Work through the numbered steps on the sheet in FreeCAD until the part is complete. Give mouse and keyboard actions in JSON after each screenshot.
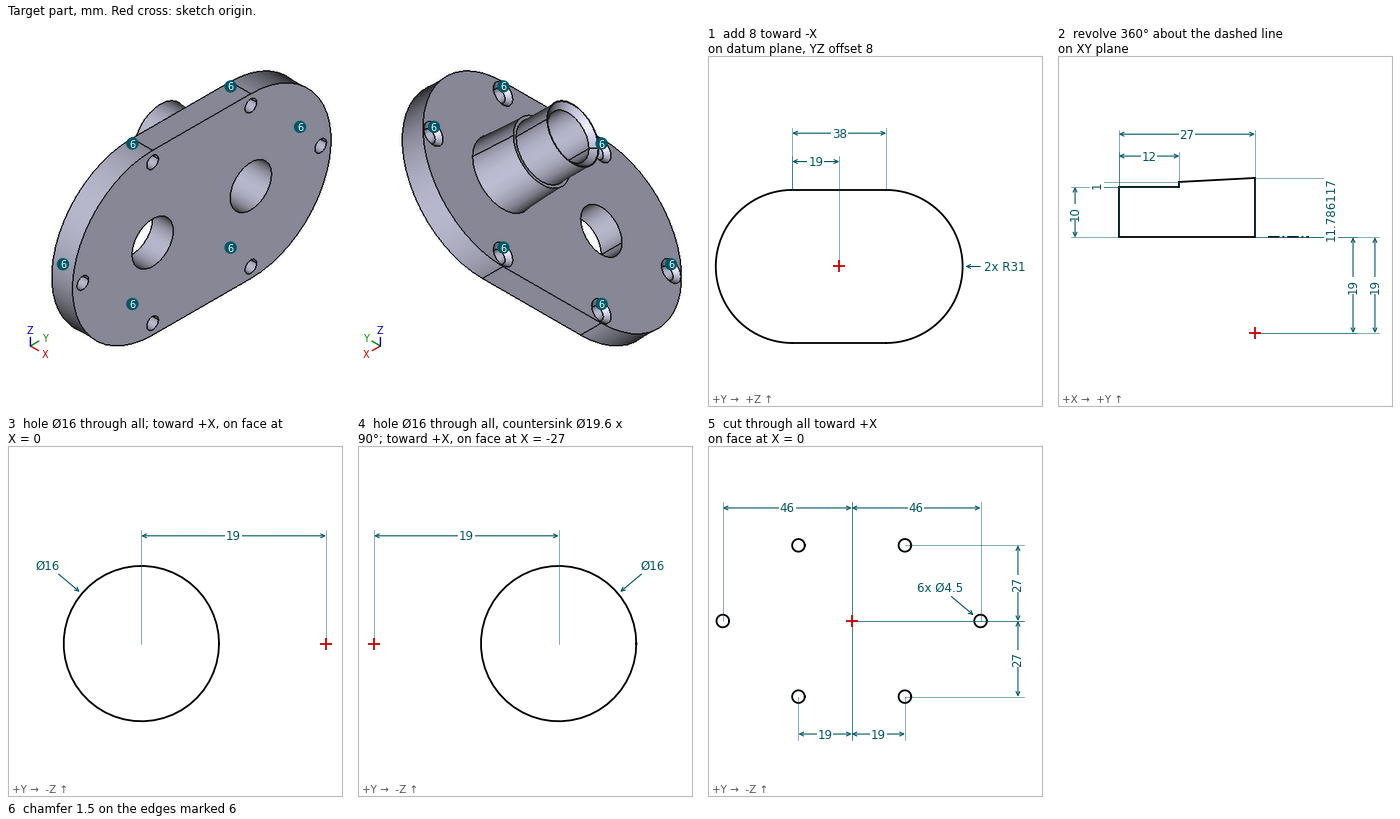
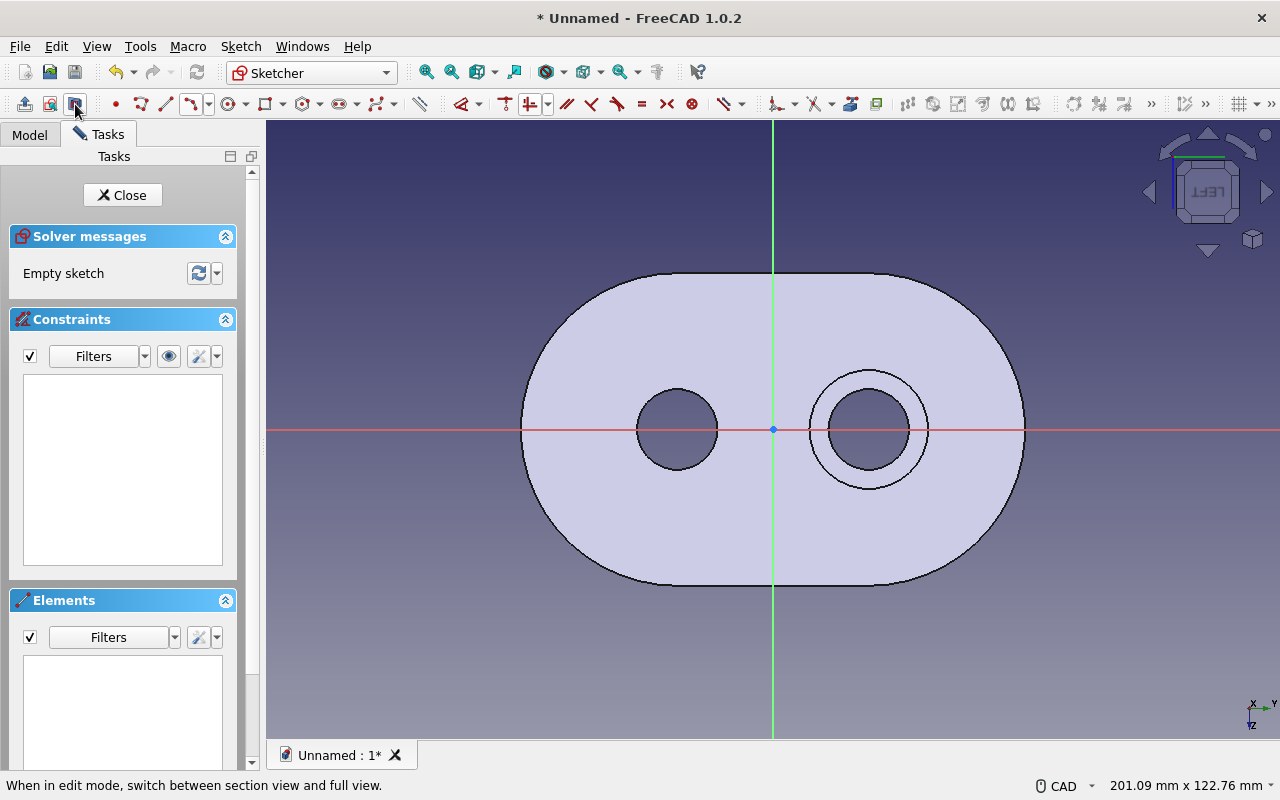
{"action": "left_click", "coordinate": [228, 104]}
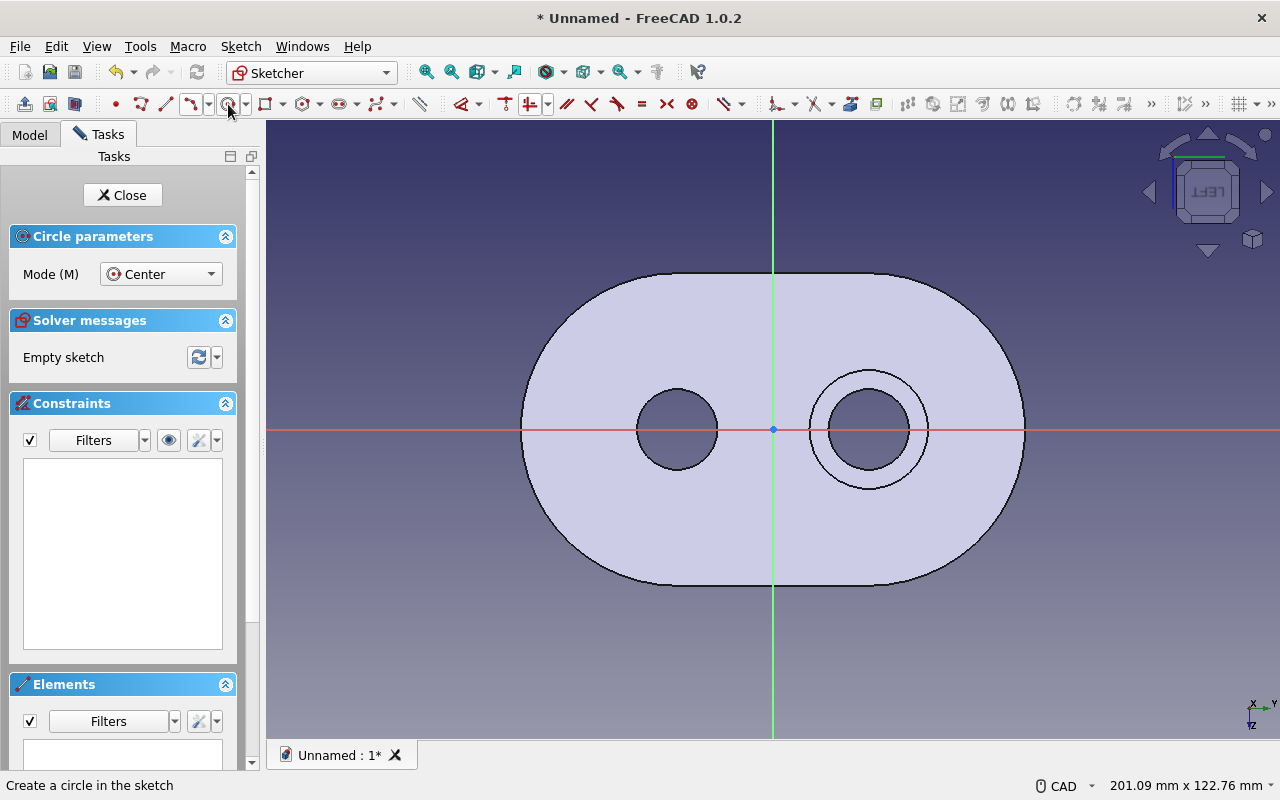
{"action": "scroll", "coordinate": [1005, 429], "scroll_direction": "up", "scroll_amount": 4}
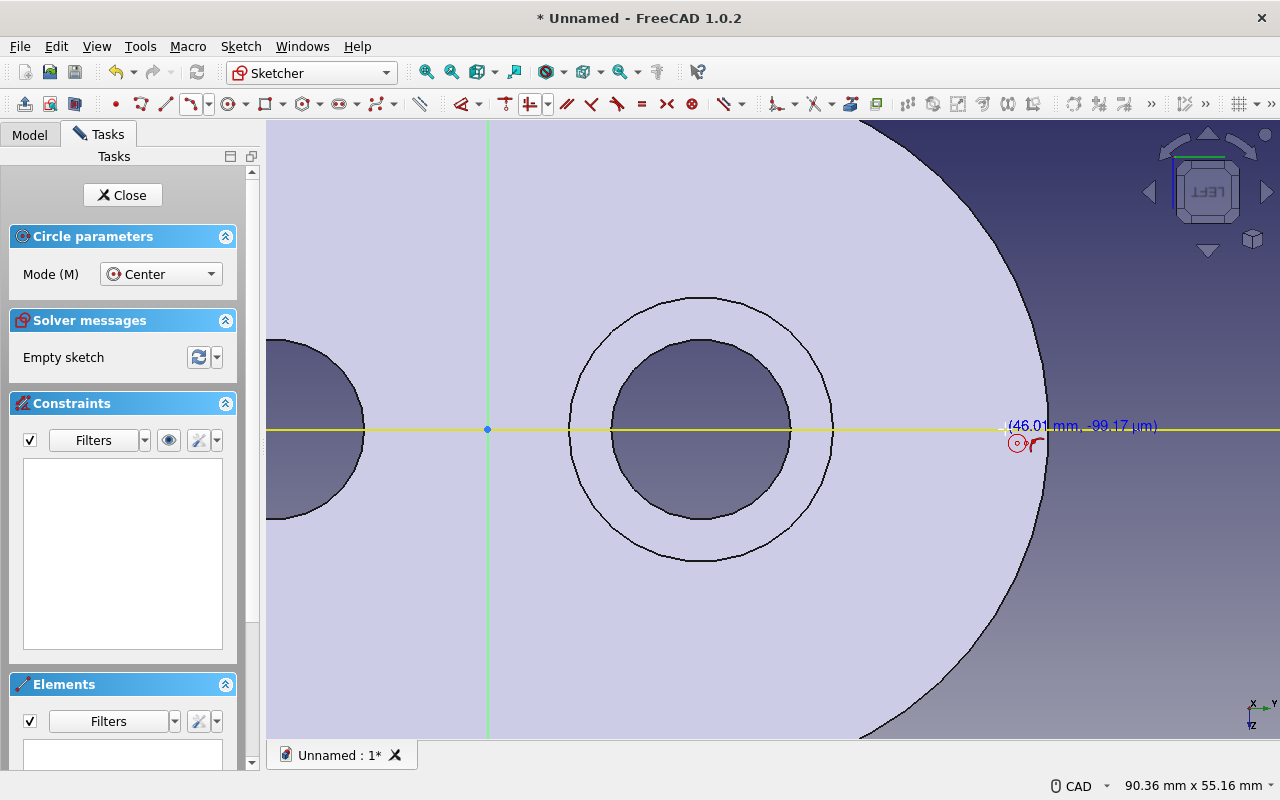
{"action": "left_click", "coordinate": [1004, 429]}
{"action": "left_click", "coordinate": [1022, 412]}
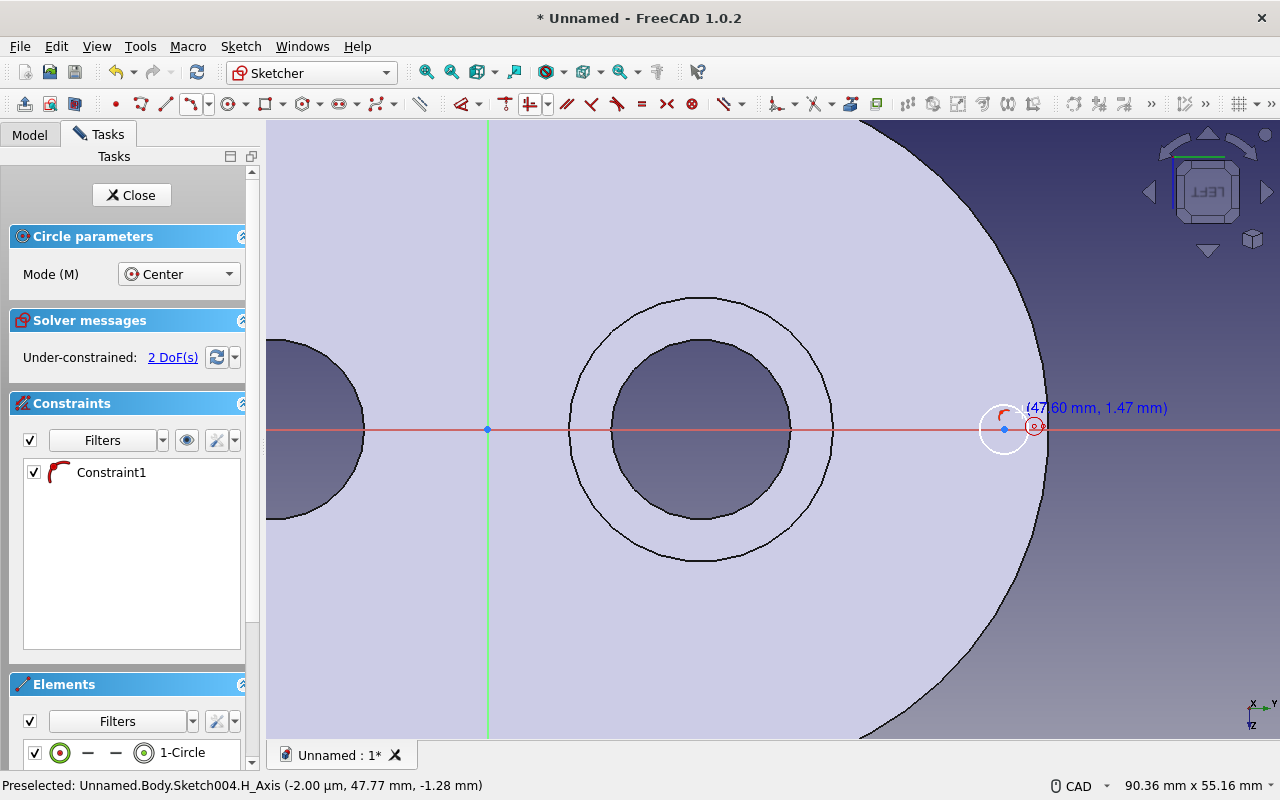
{"action": "scroll", "coordinate": [968, 430], "scroll_direction": "down", "scroll_amount": 3}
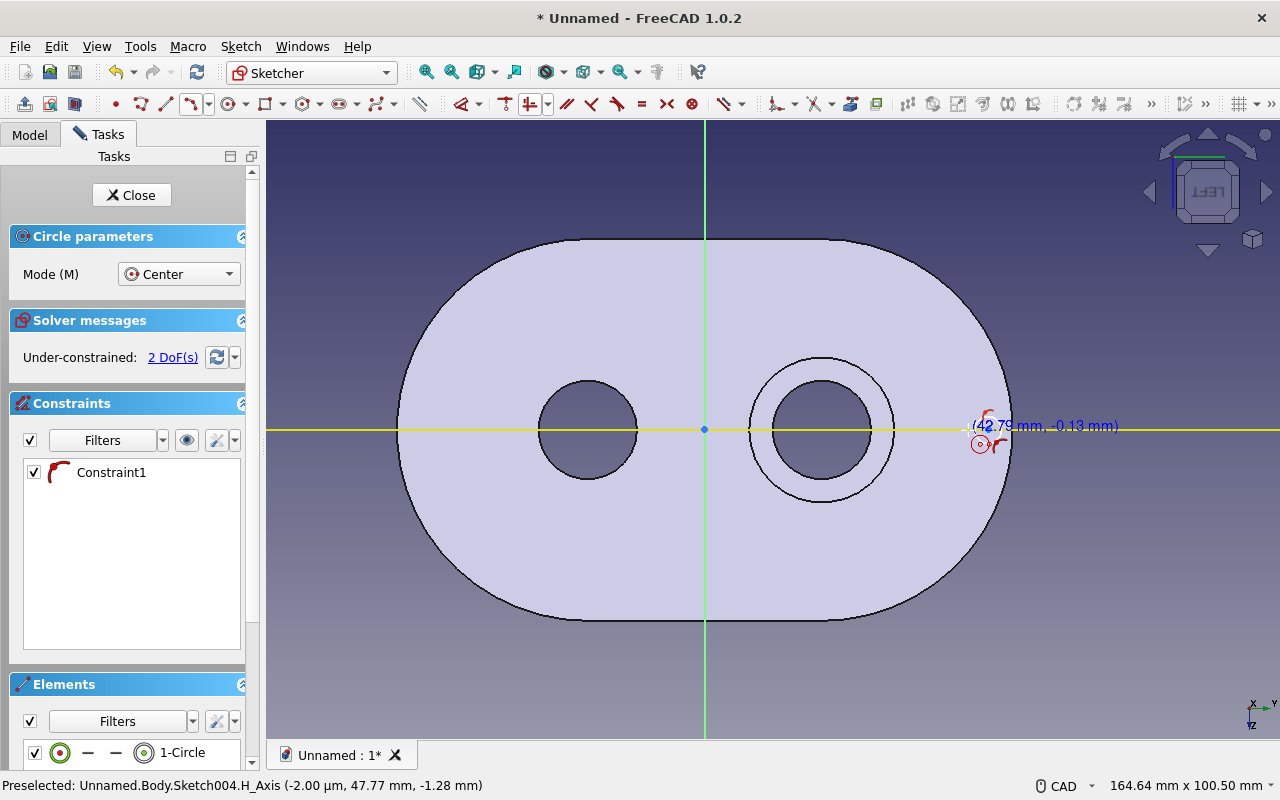
{"action": "scroll", "coordinate": [822, 596], "scroll_direction": "up", "scroll_amount": 3}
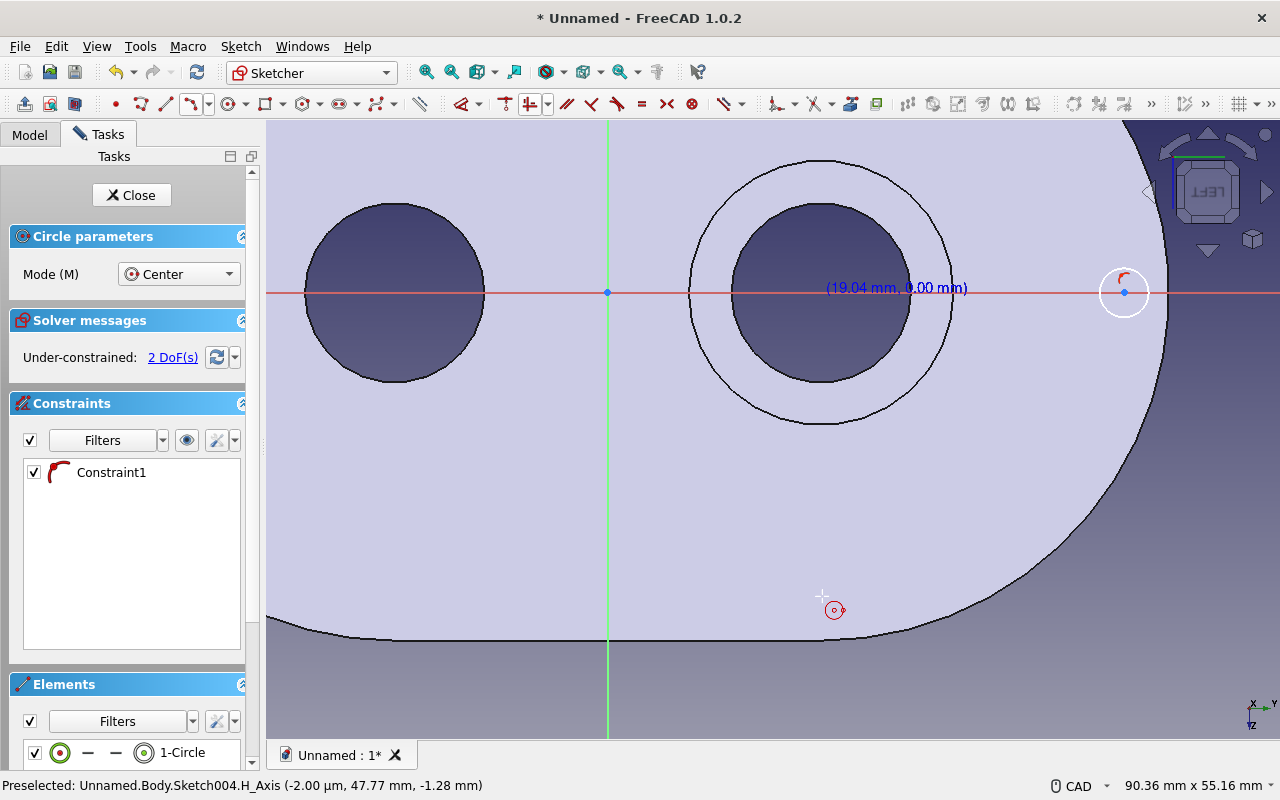
{"action": "left_click", "coordinate": [821, 596]}
{"action": "left_click", "coordinate": [839, 578]}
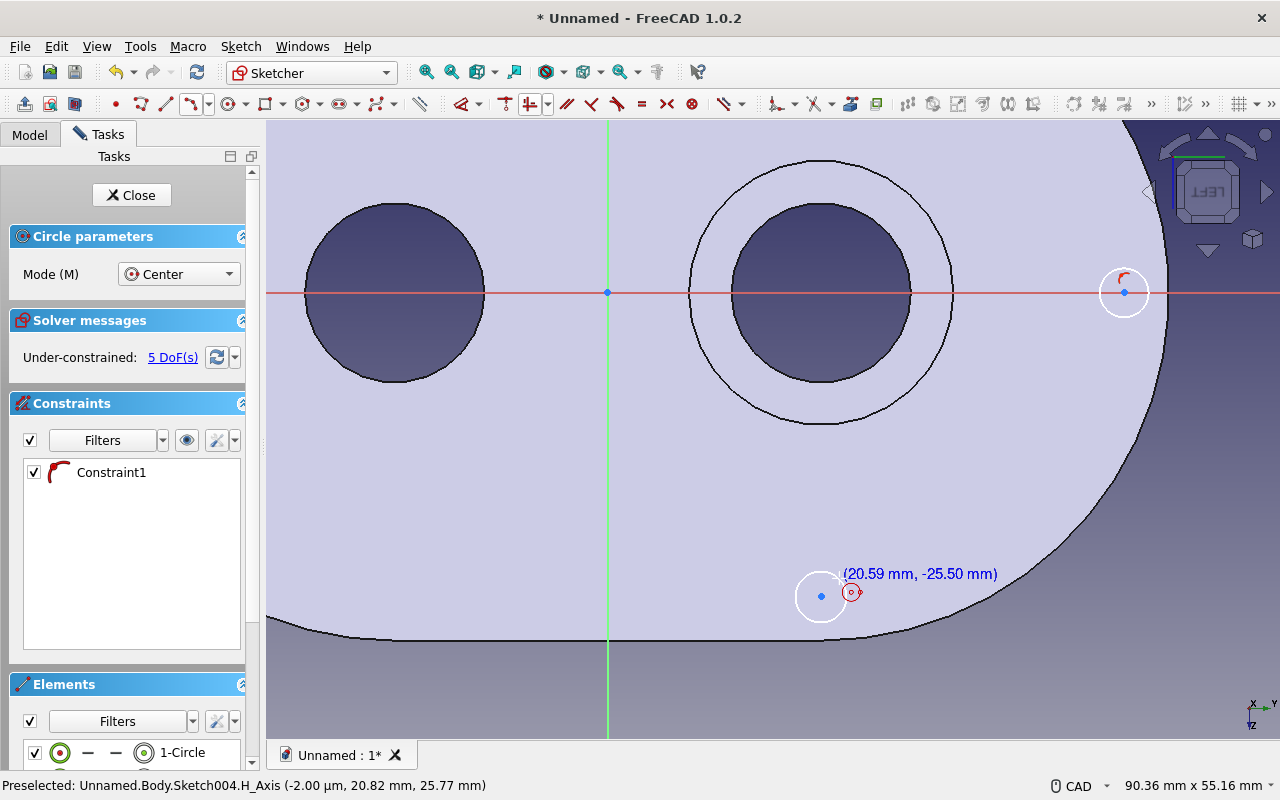
{"action": "scroll", "coordinate": [822, 596], "scroll_direction": "down", "scroll_amount": 3}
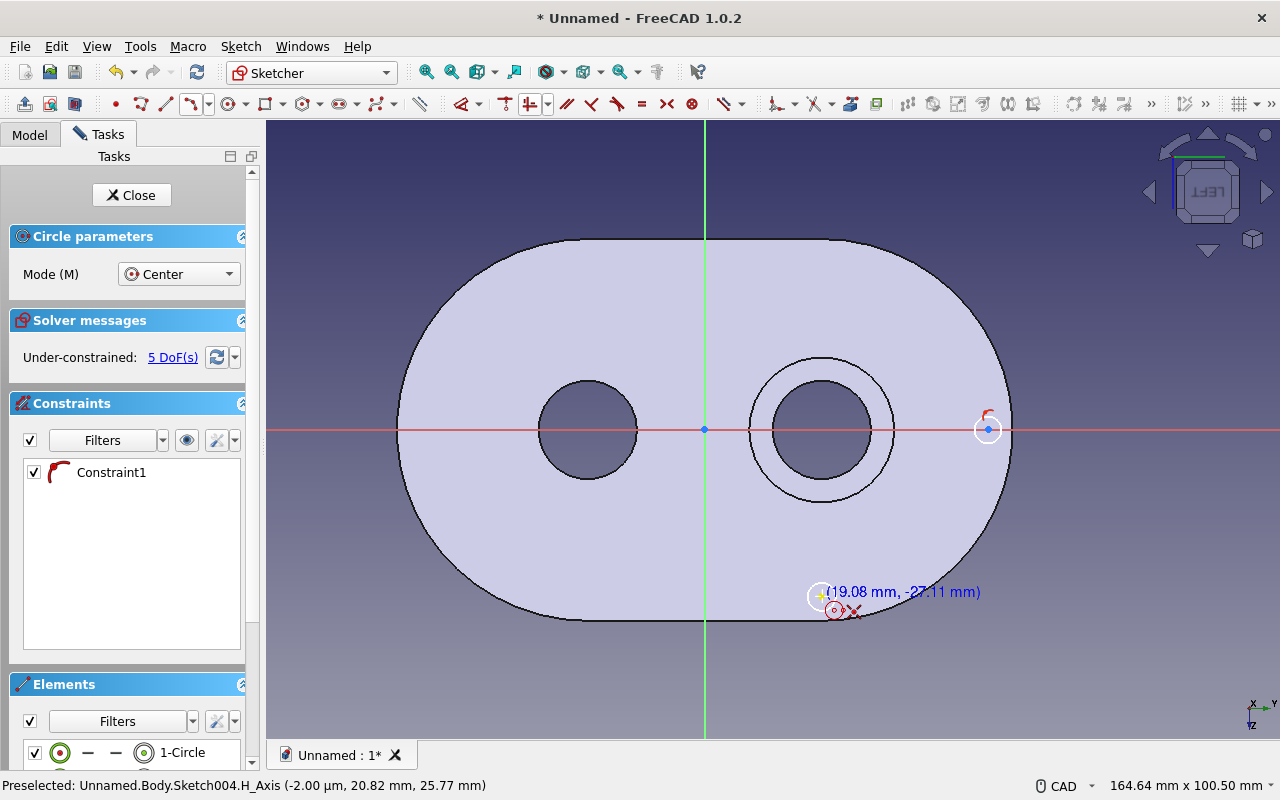
{"action": "scroll", "coordinate": [822, 264], "scroll_direction": "up", "scroll_amount": 3}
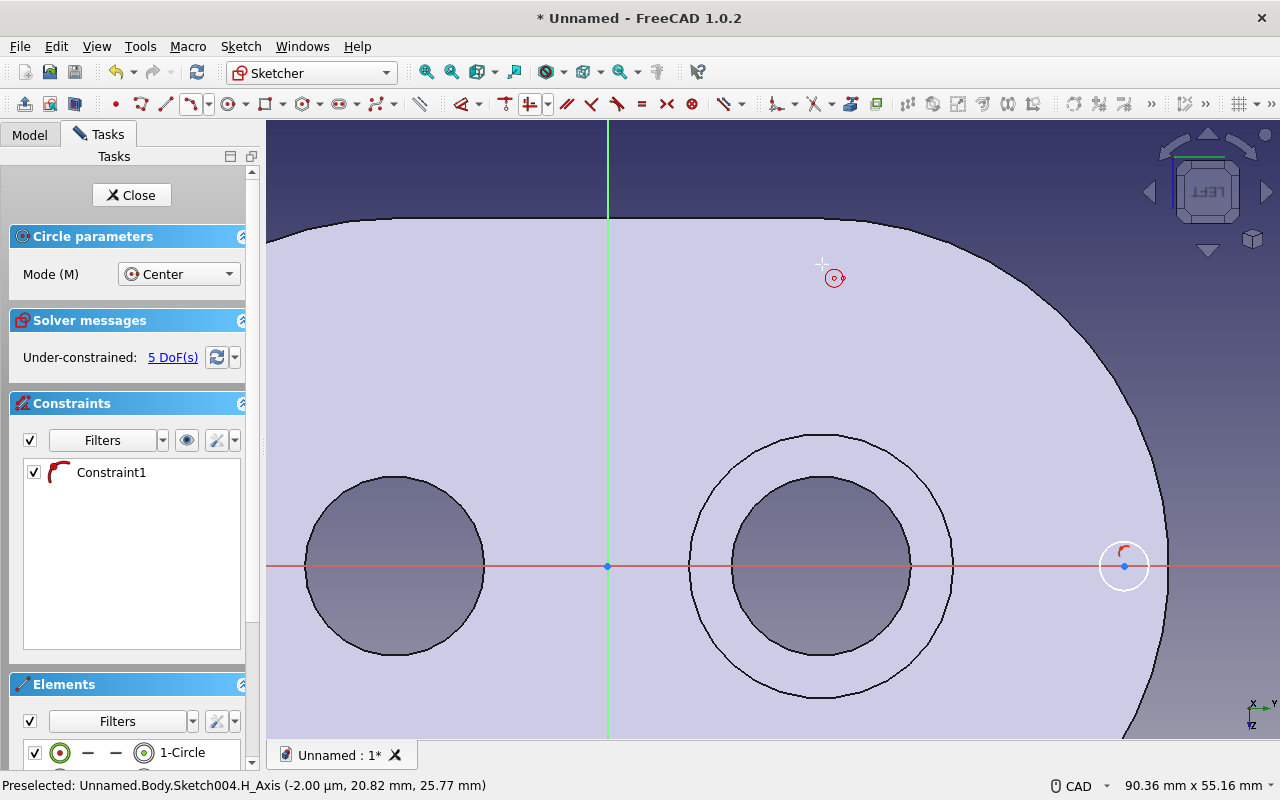
{"action": "left_click", "coordinate": [821, 263]}
{"action": "left_click", "coordinate": [839, 245]}